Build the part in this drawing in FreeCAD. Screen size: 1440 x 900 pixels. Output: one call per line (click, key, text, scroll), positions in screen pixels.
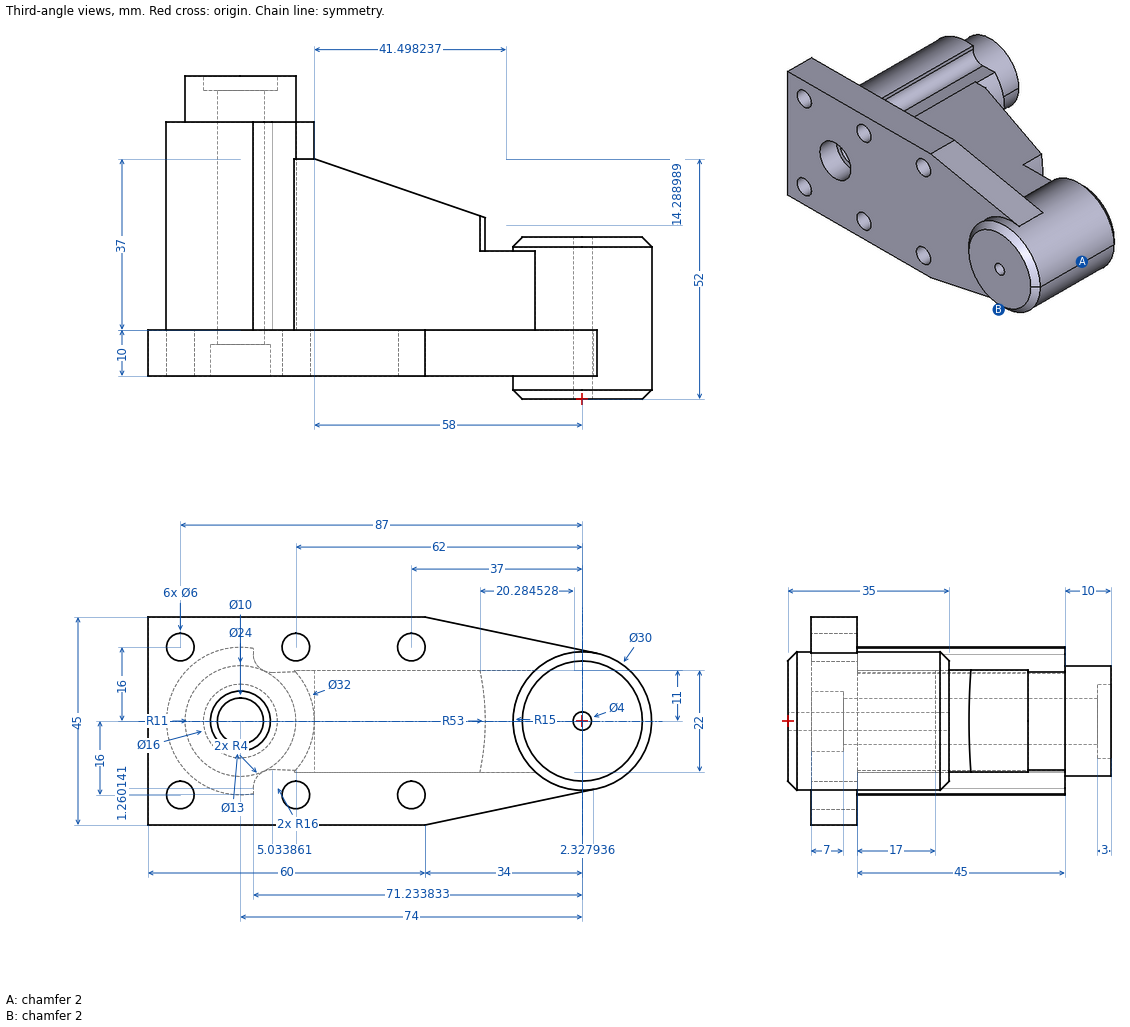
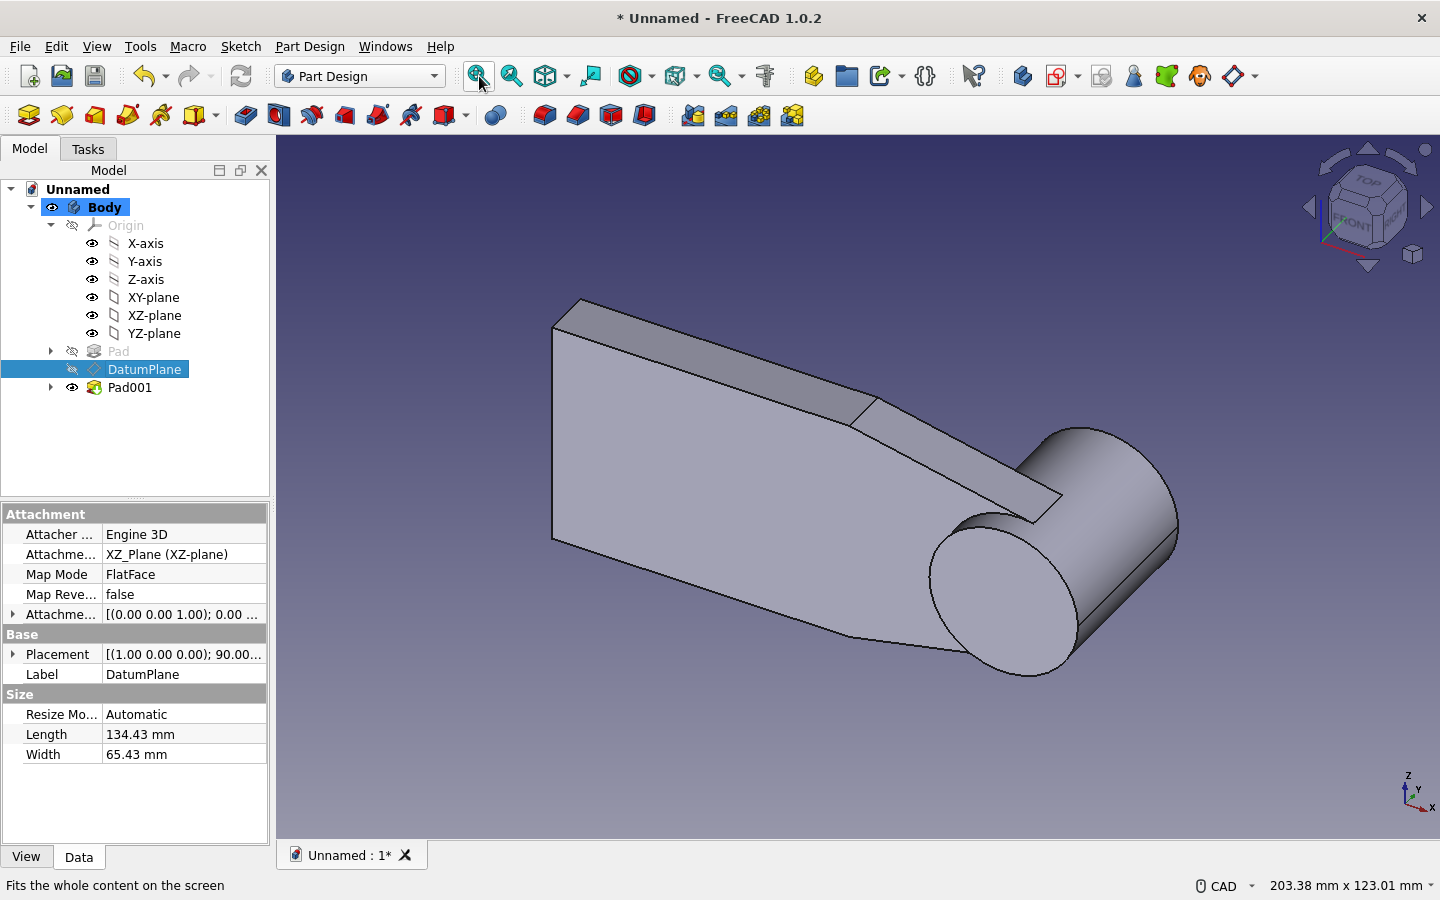
key(4)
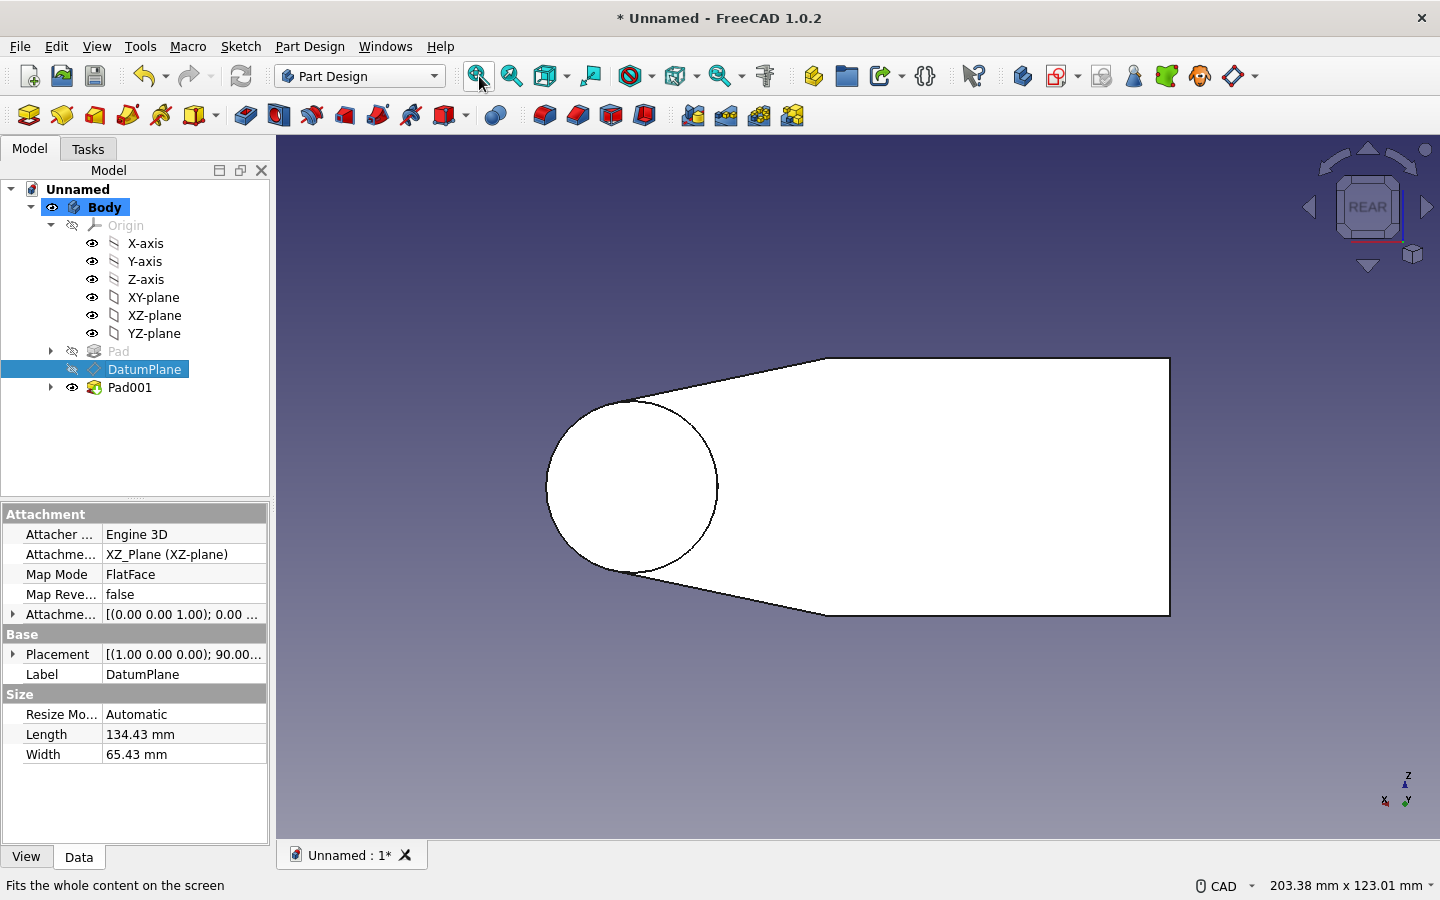
click(892, 486)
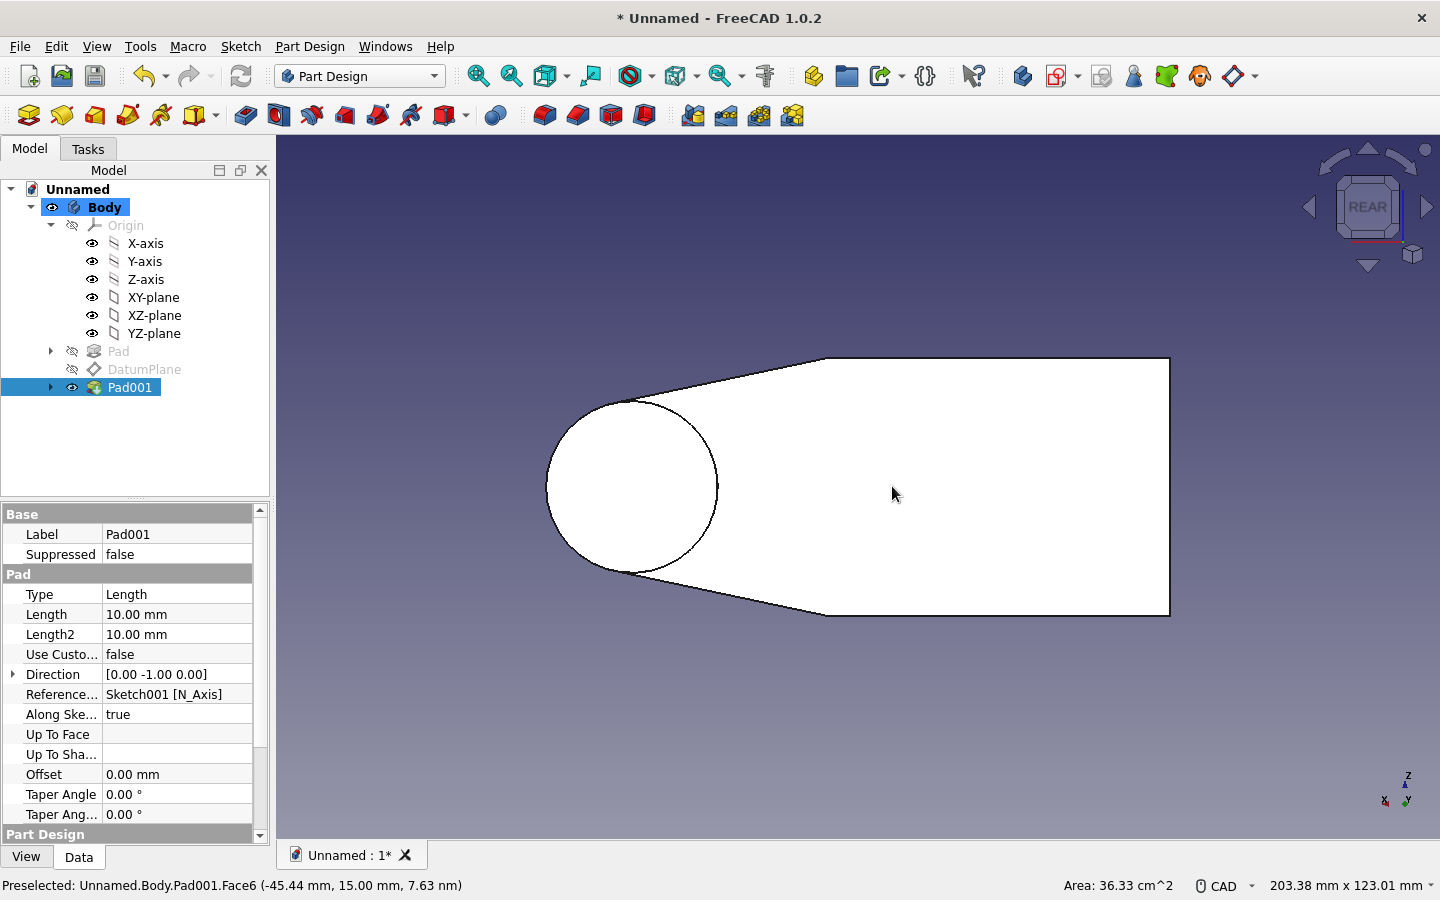
click(1056, 76)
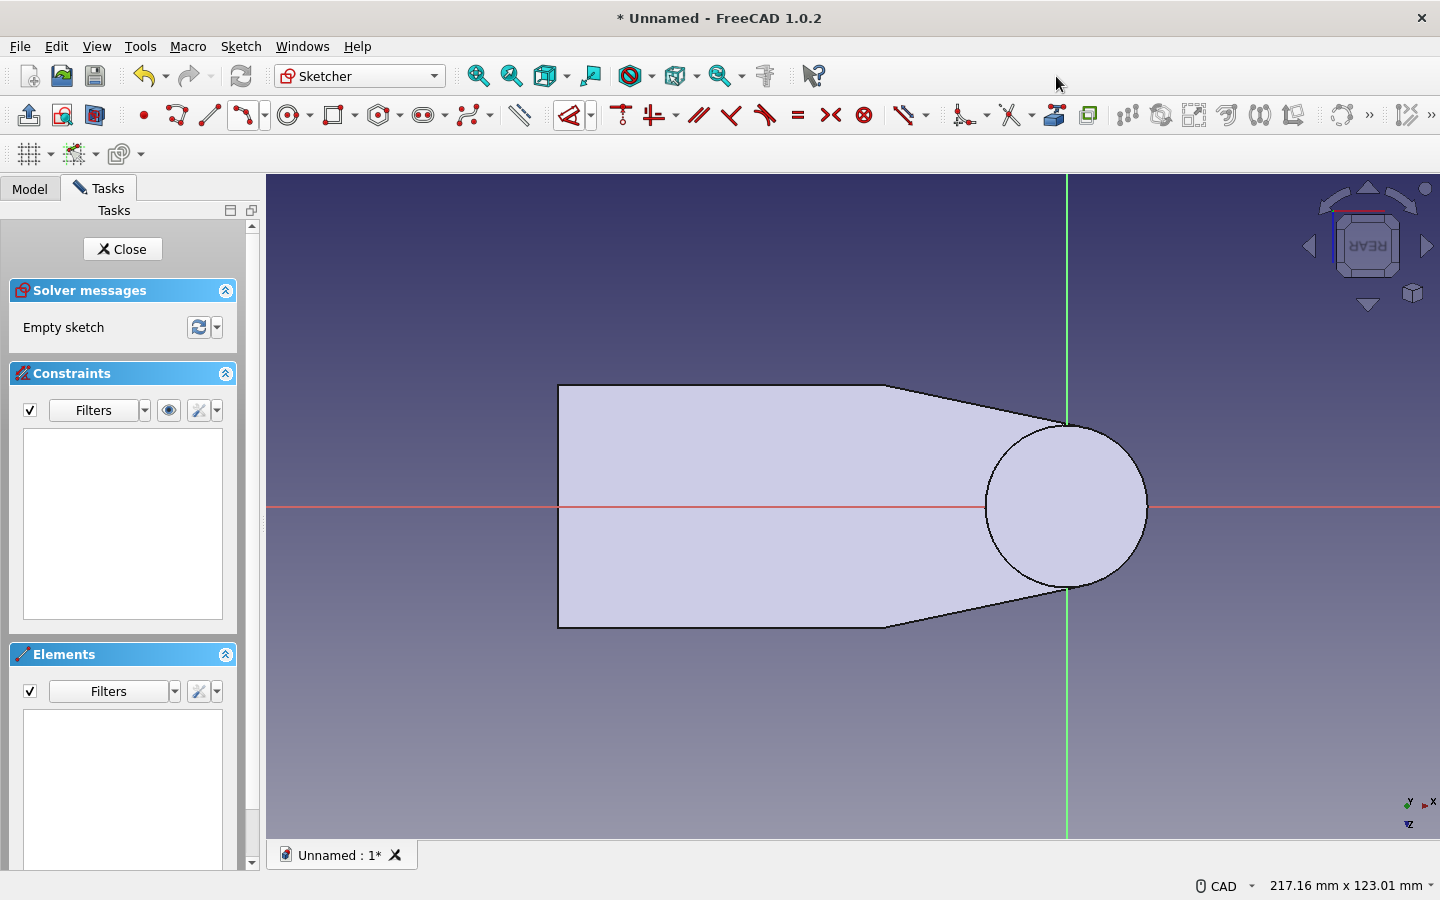
click(95, 116)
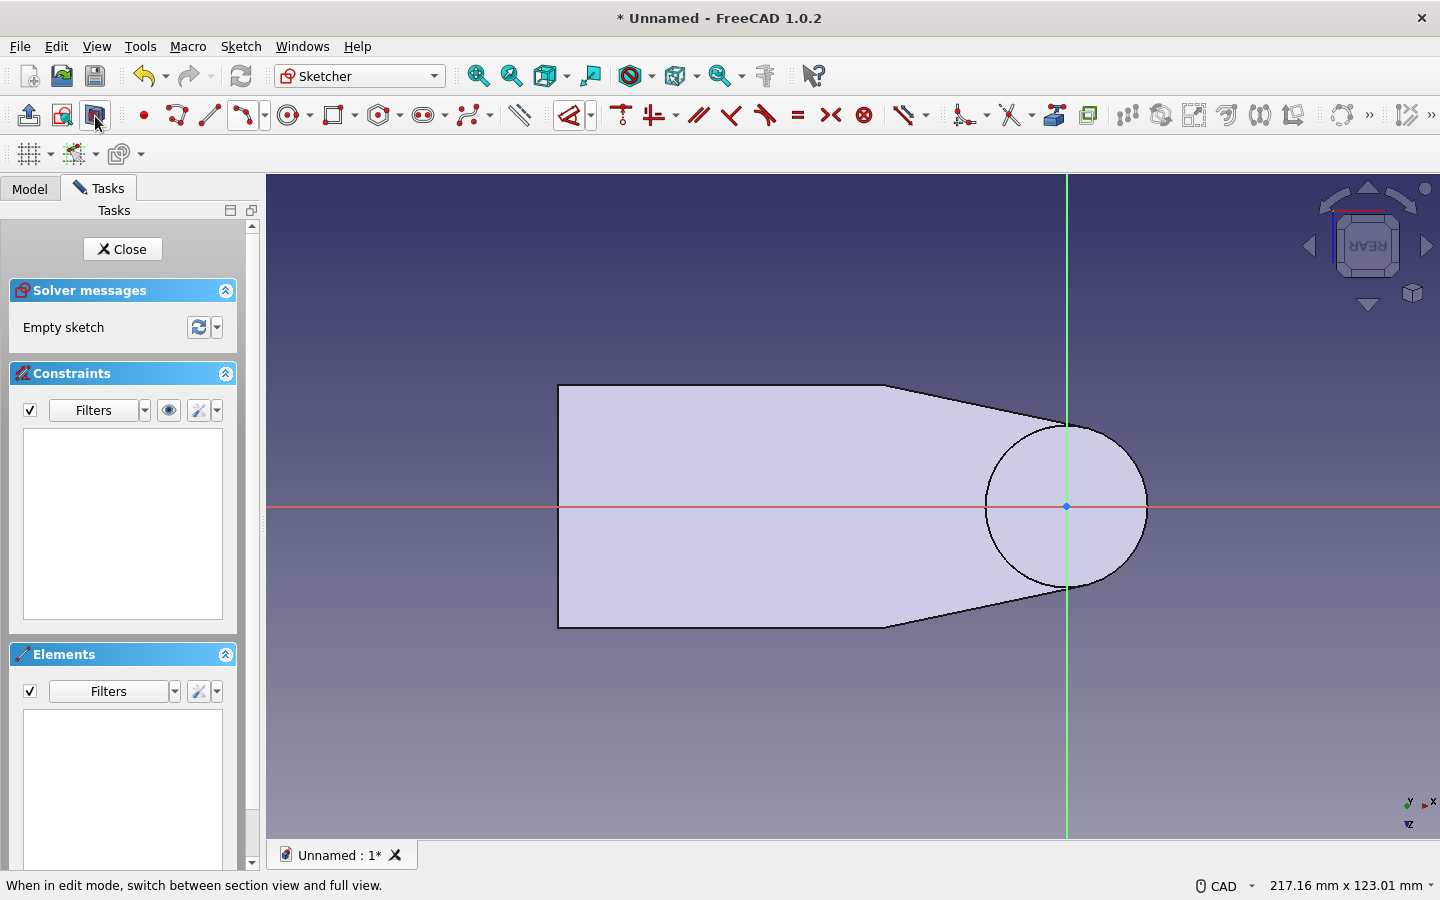
scroll(598, 506, up, 5)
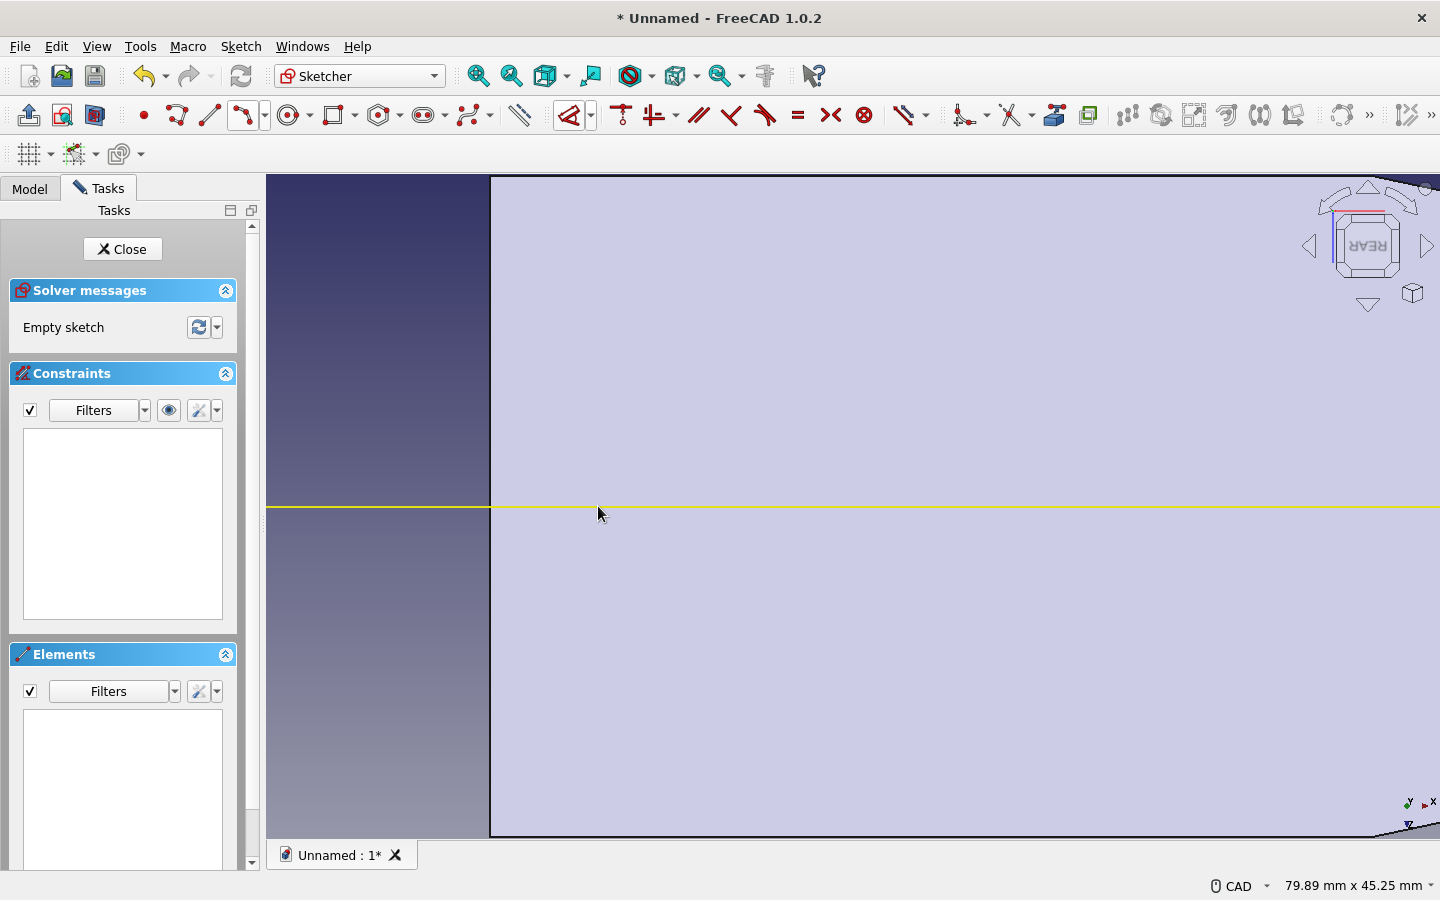
click(288, 116)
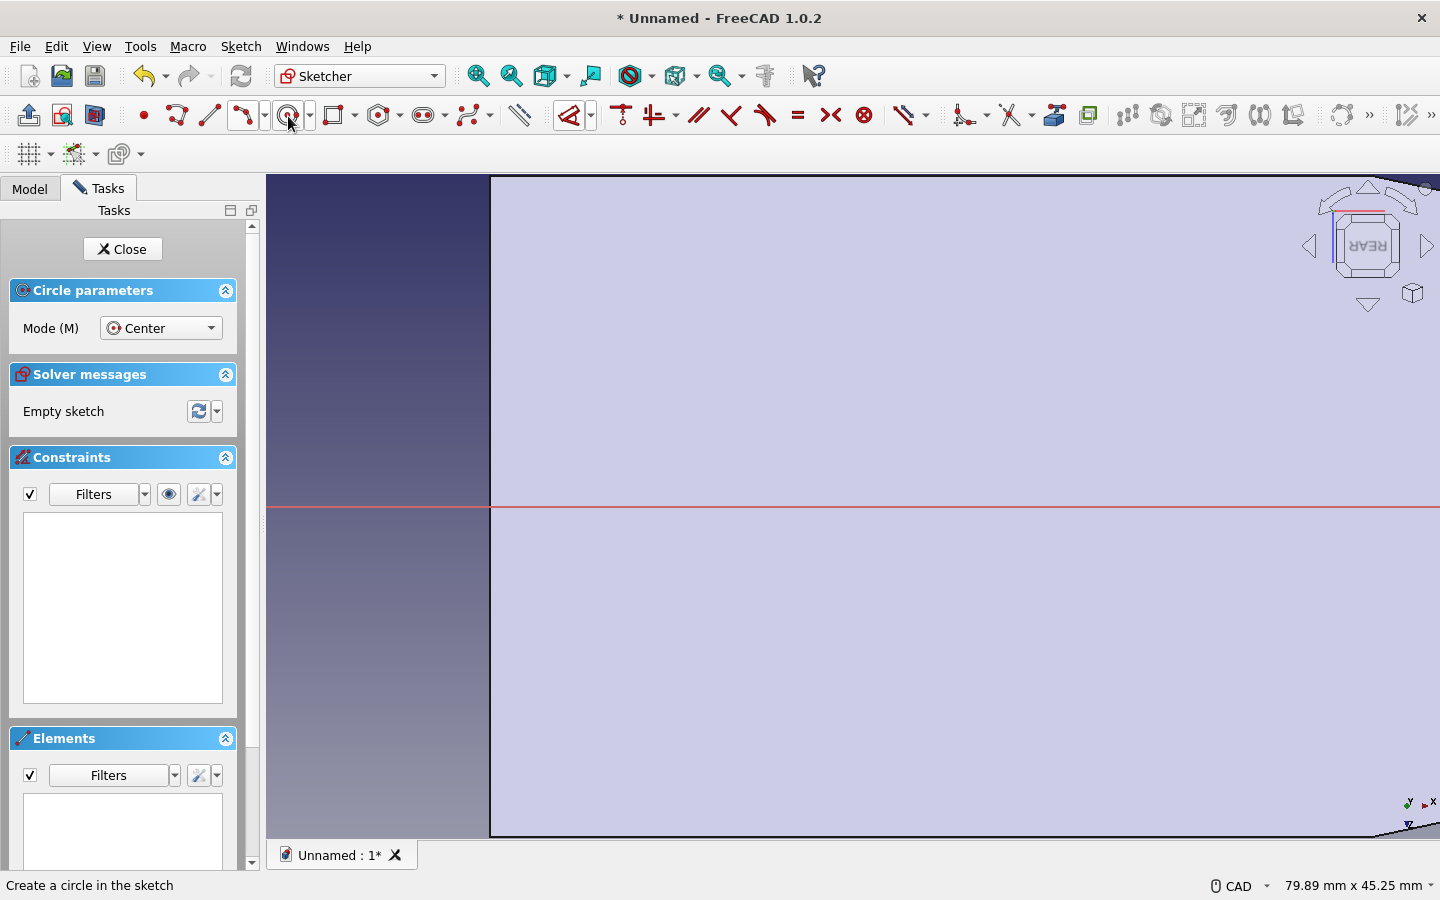
click(784, 506)
click(950, 340)
key(Escape)